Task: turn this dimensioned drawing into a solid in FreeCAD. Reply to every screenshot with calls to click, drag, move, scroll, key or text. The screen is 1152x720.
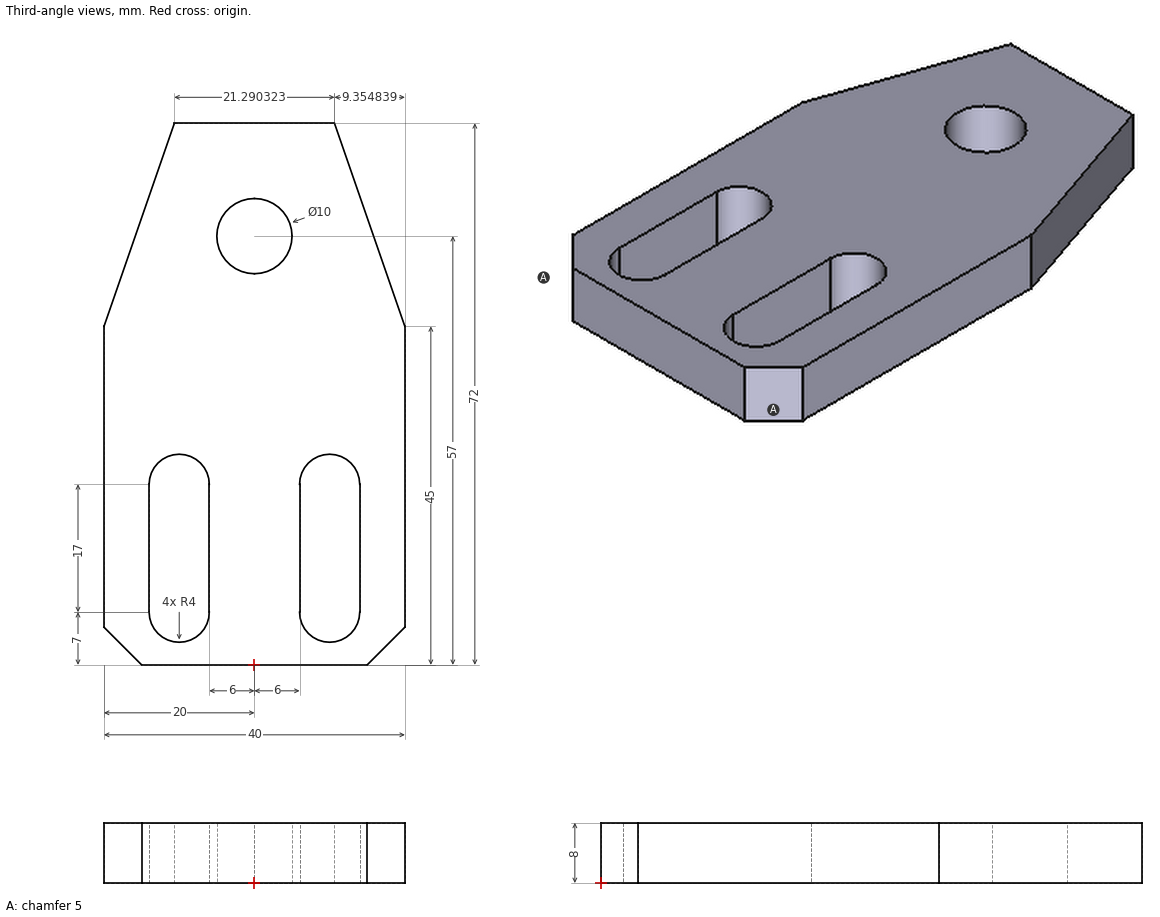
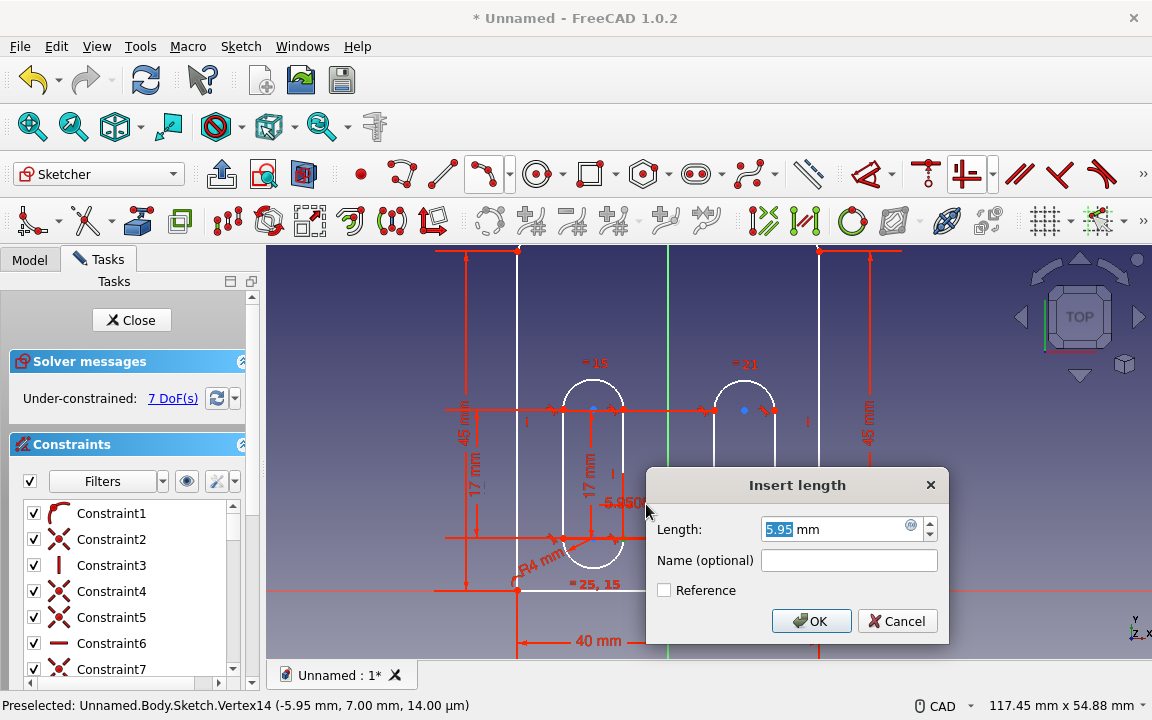
text(6)
key(Return)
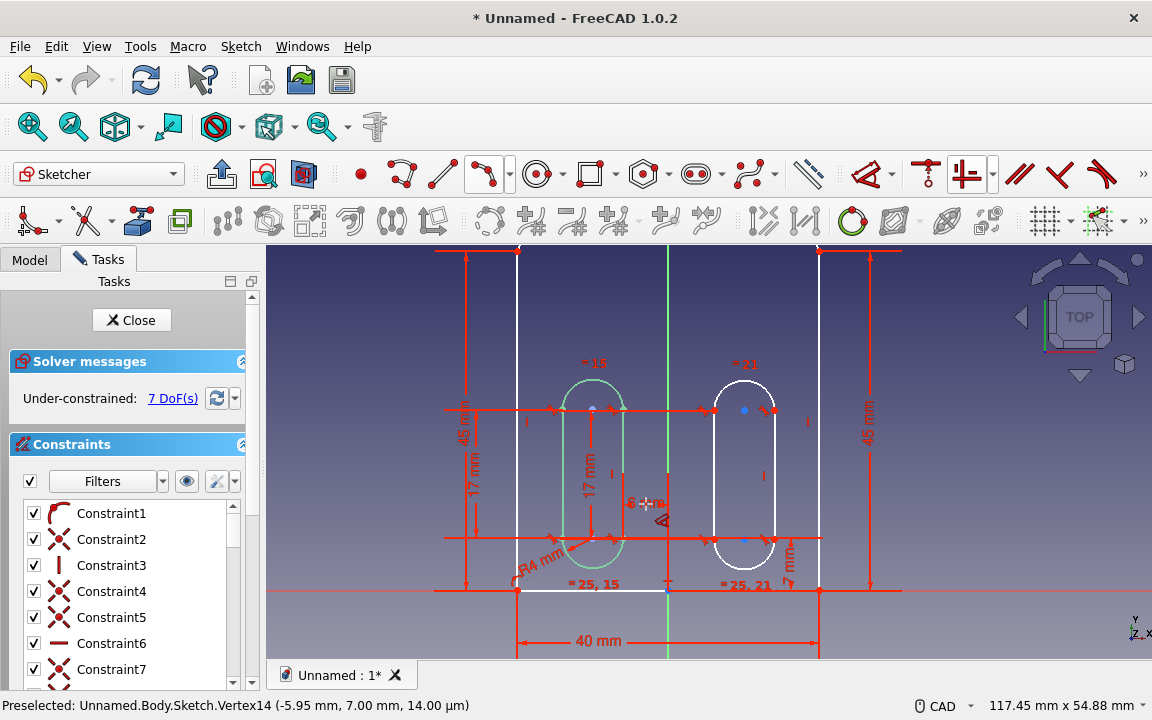
click(714, 539)
click(691, 625)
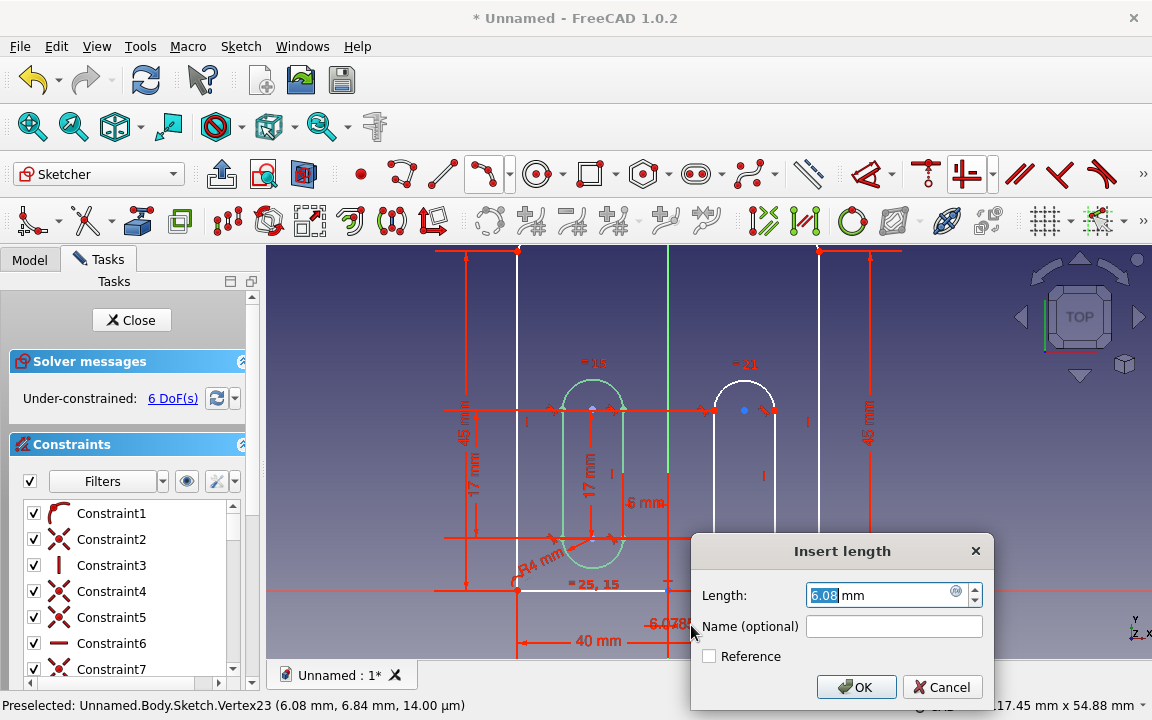
text(6)
key(Return)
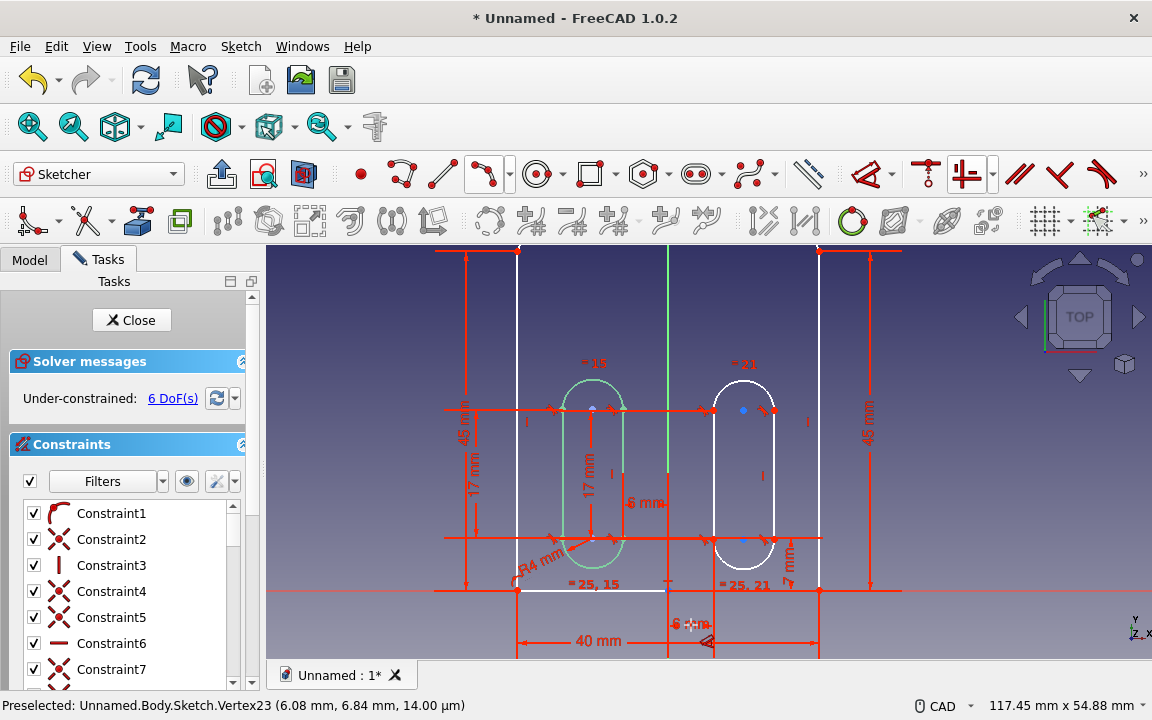
click(714, 539)
click(634, 565)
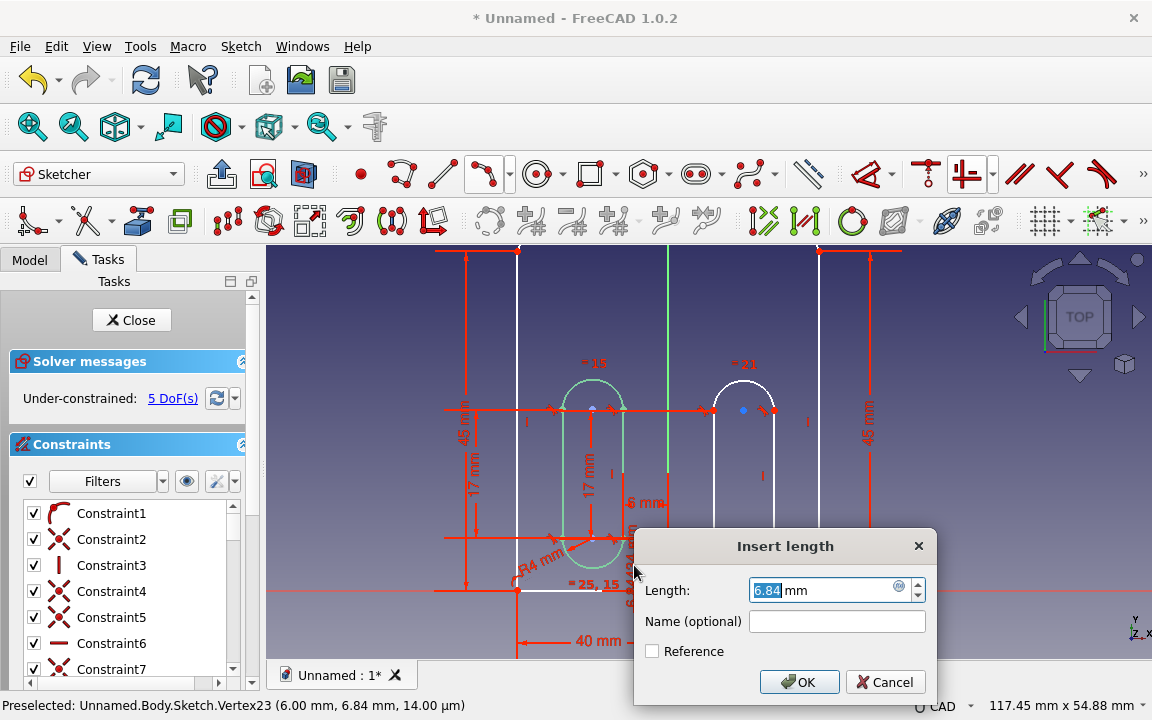
text(7)
key(Return)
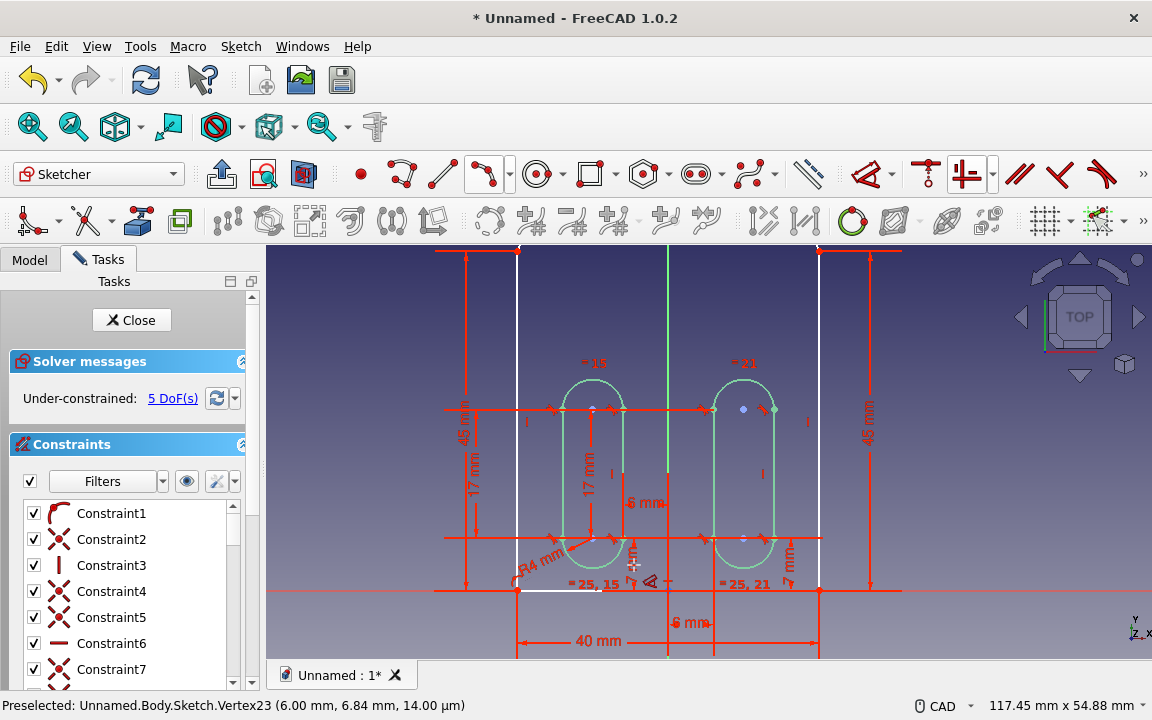
scroll(618, 560, down, 4)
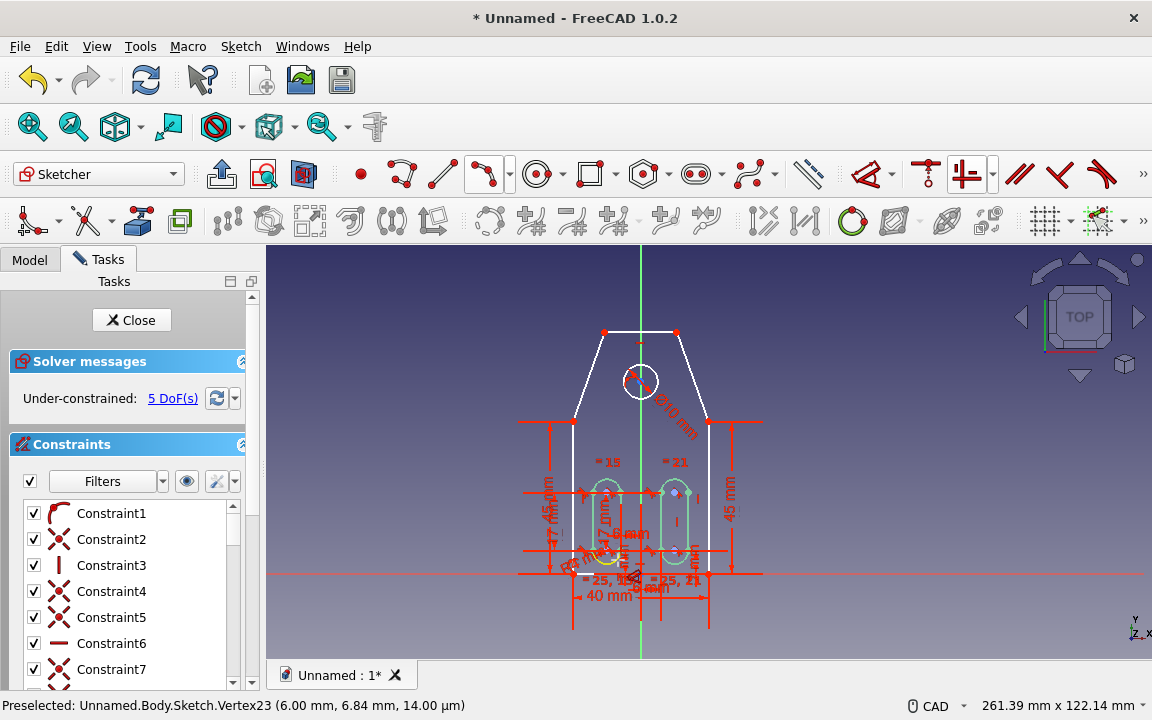
click(641, 382)
click(723, 478)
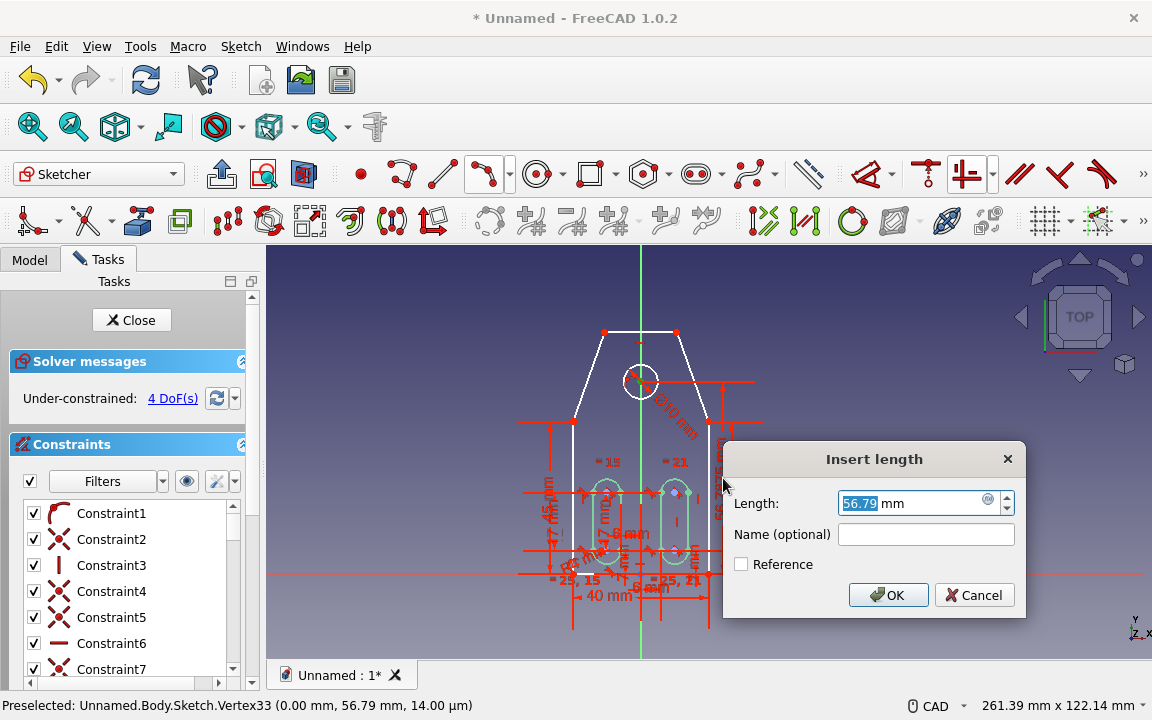
text(57)
key(Return)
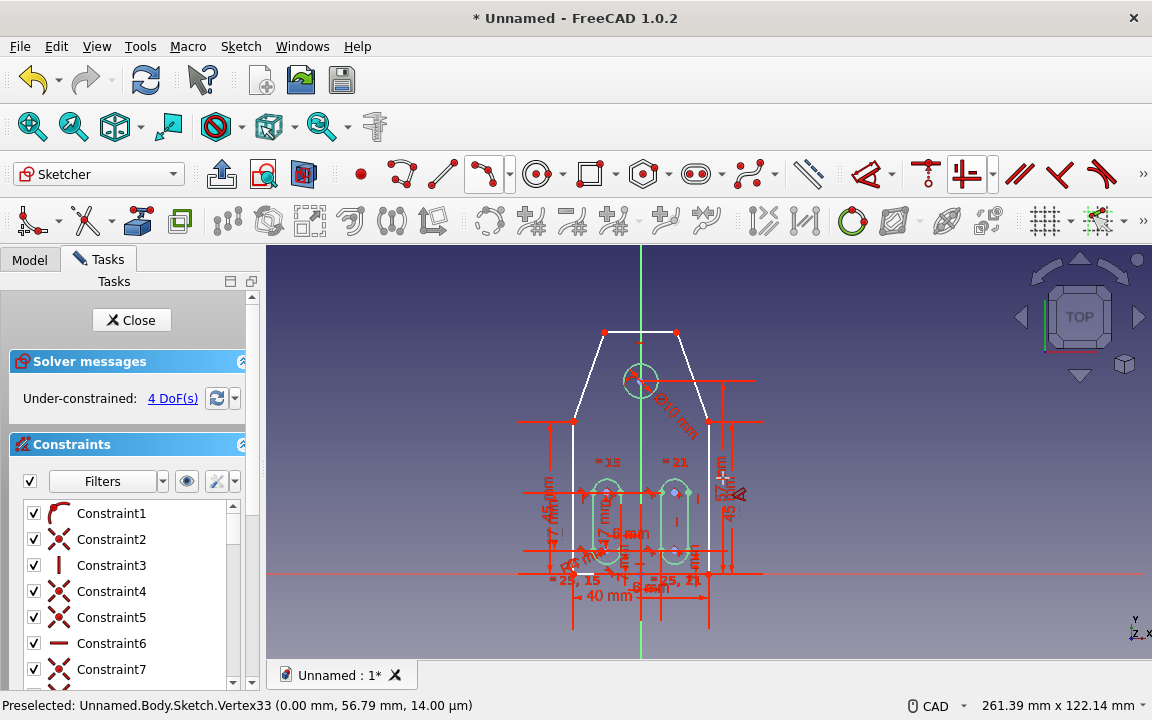
click(573, 574)
click(591, 468)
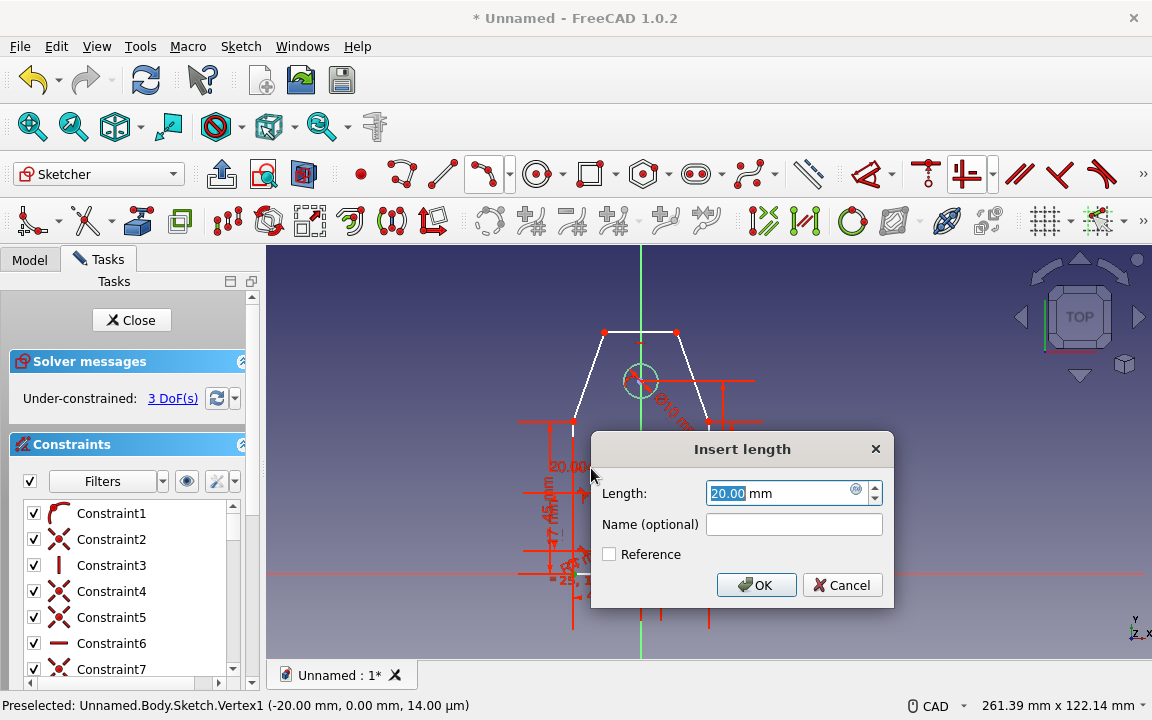
text(20)
key(Return)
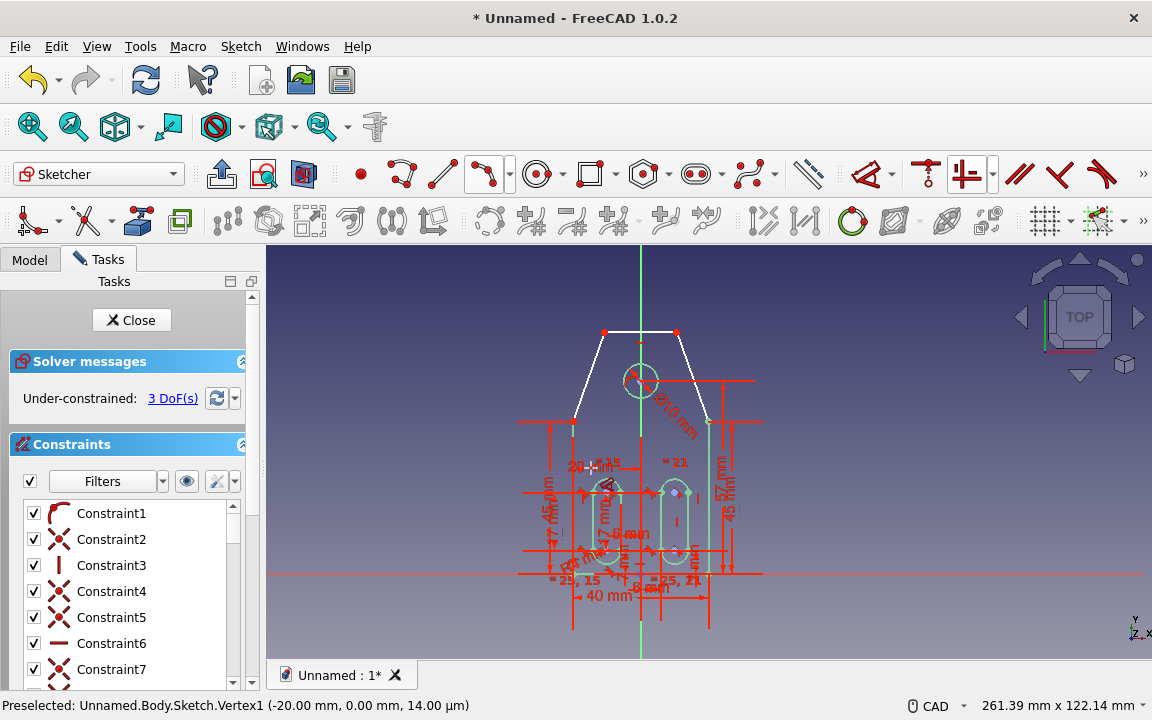
click(677, 332)
click(711, 368)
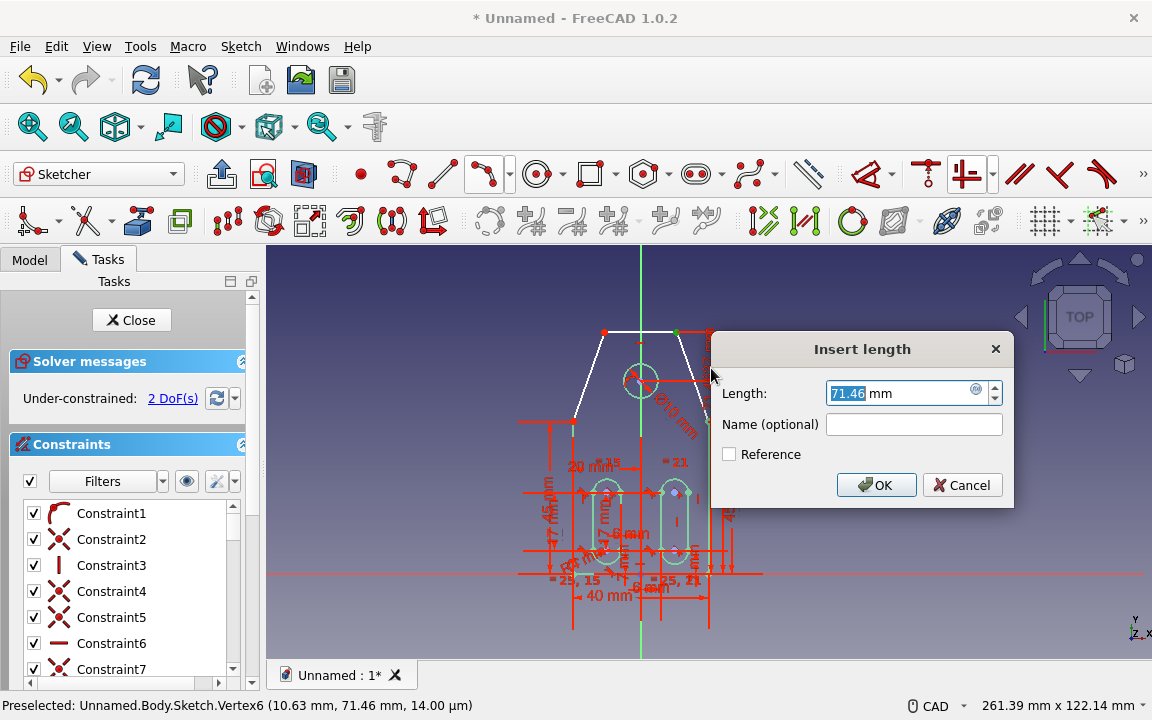
text(72)
key(Return)